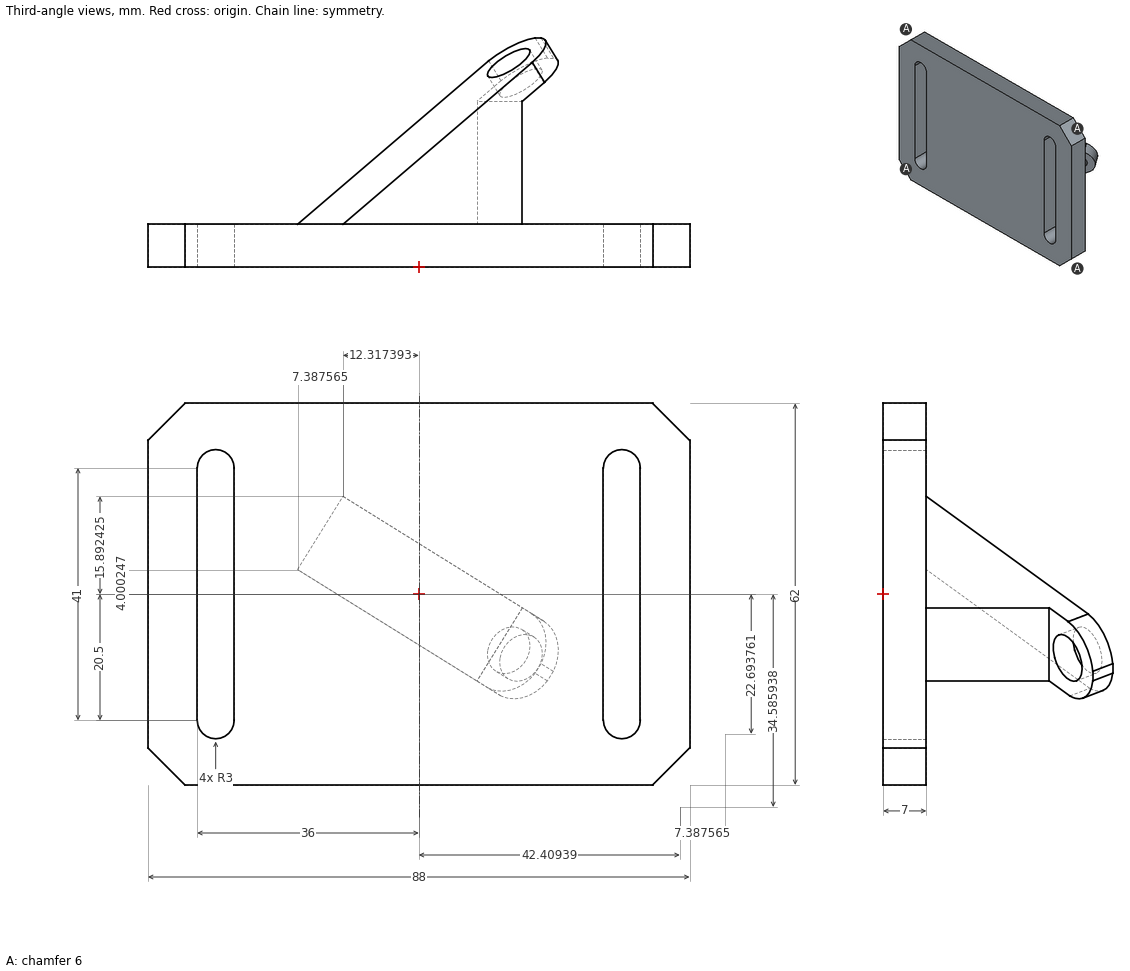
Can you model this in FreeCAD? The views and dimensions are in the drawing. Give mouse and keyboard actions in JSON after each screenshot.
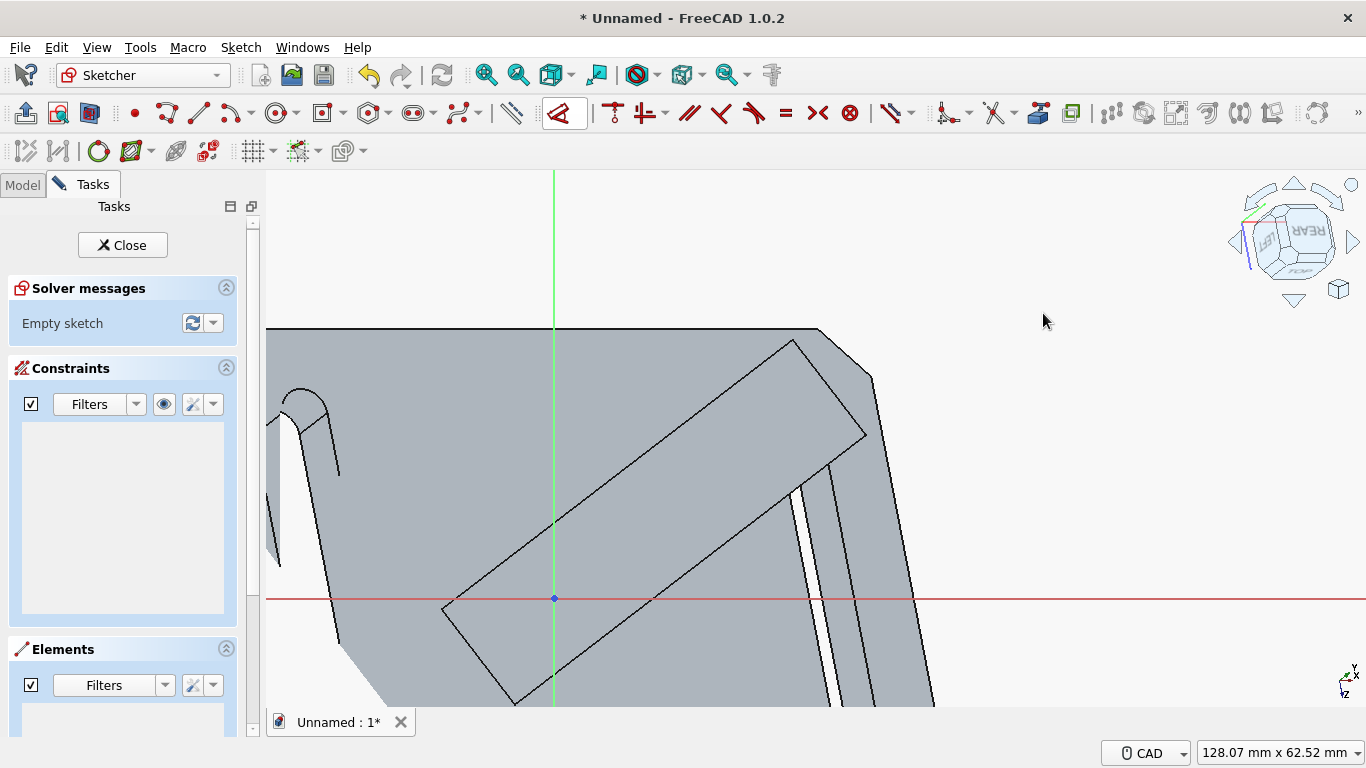
{"action": "left_click", "coordinate": [168, 114]}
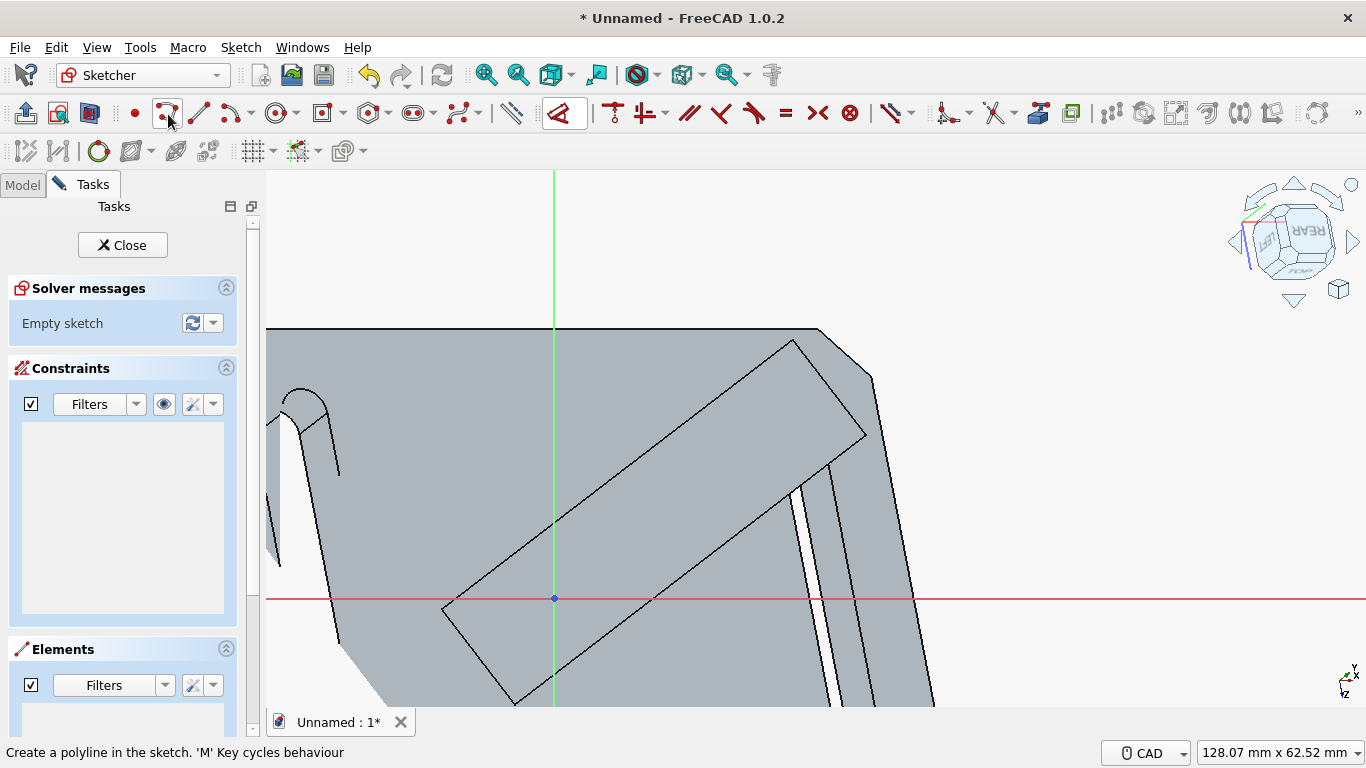
{"action": "left_click", "coordinate": [819, 471]}
{"action": "left_click", "coordinate": [856, 453]}
{"action": "left_click", "coordinate": [939, 464]}
{"action": "left_click", "coordinate": [772, 277]}
{"action": "left_click", "coordinate": [741, 379]}
{"action": "right_click", "coordinate": [741, 379]}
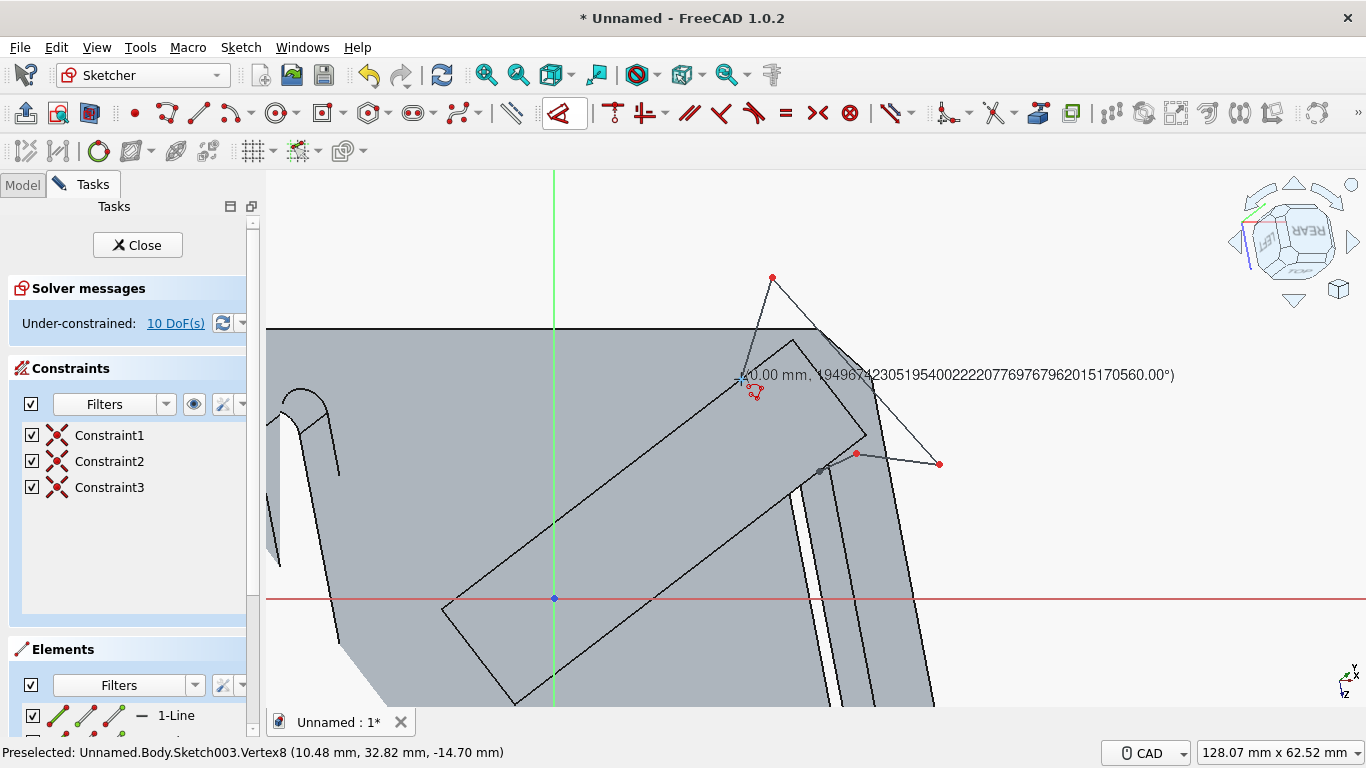
{"action": "left_click", "coordinate": [254, 114]}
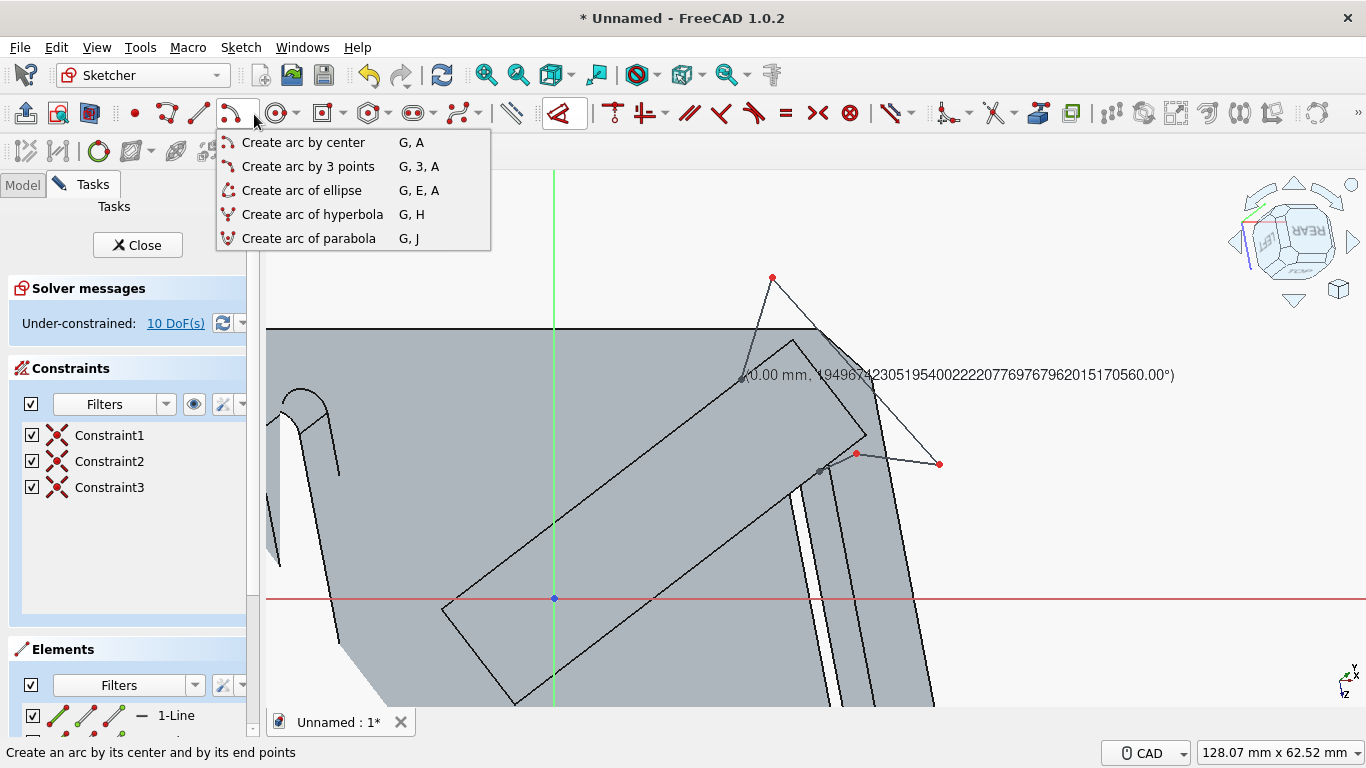
{"action": "left_click", "coordinate": [354, 166]}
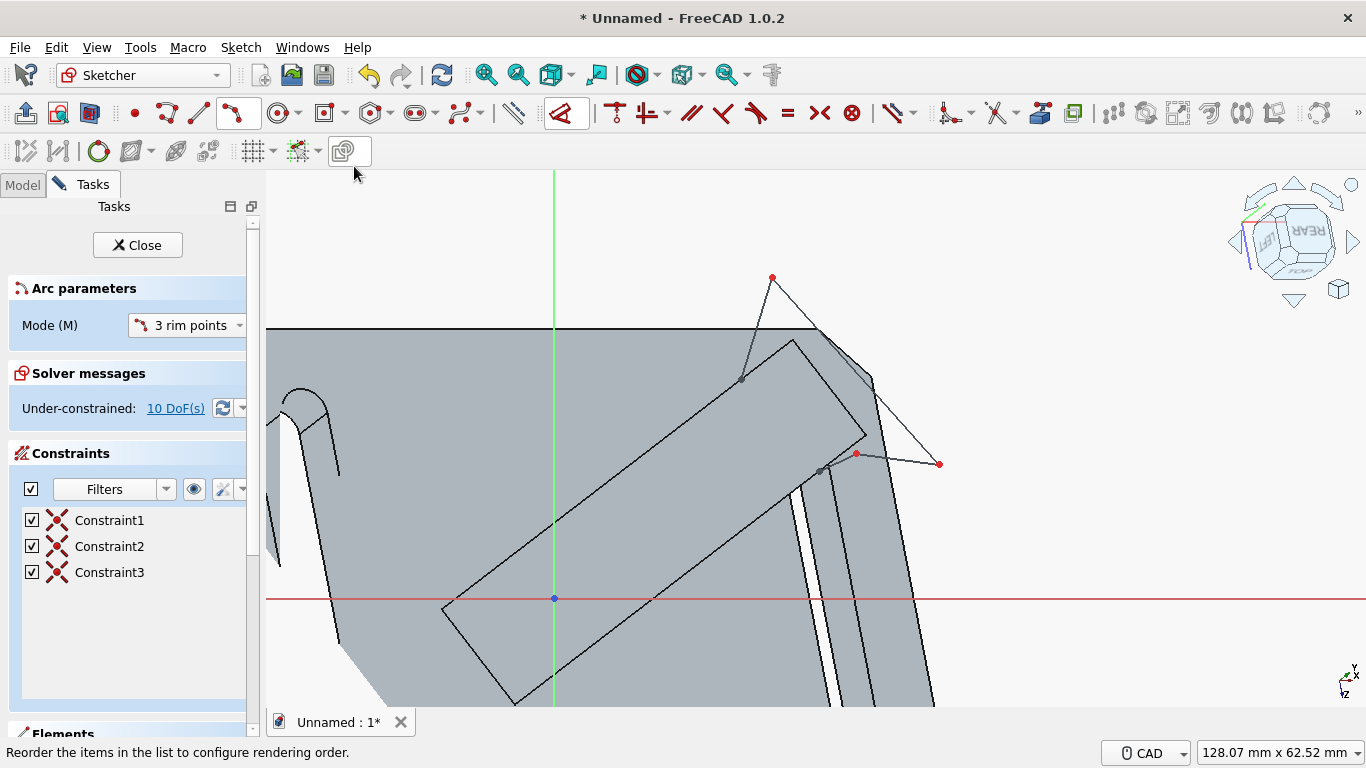
{"action": "left_click", "coordinate": [741, 380]}
{"action": "left_click", "coordinate": [819, 472]}
{"action": "left_click", "coordinate": [828, 385]}
{"action": "key", "text": "Escape"}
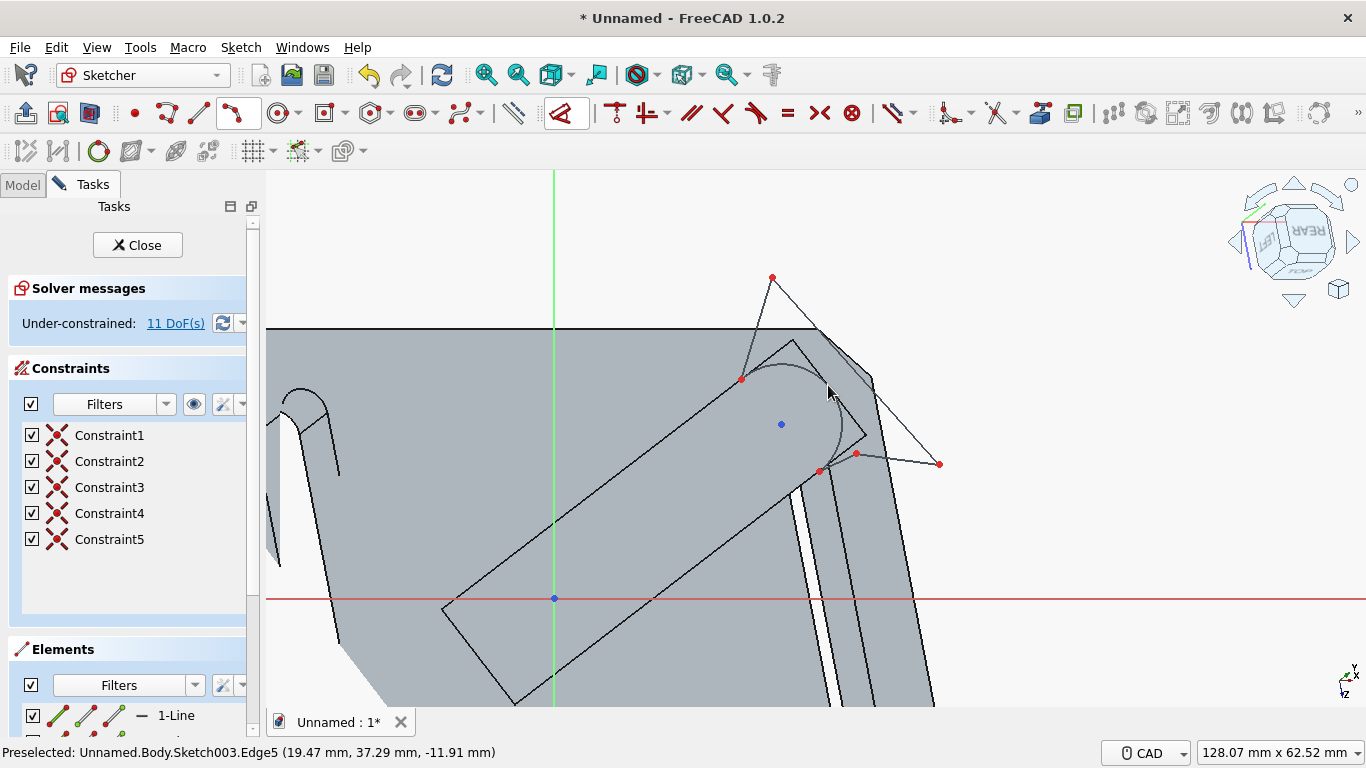
{"action": "left_click", "coordinate": [842, 421]}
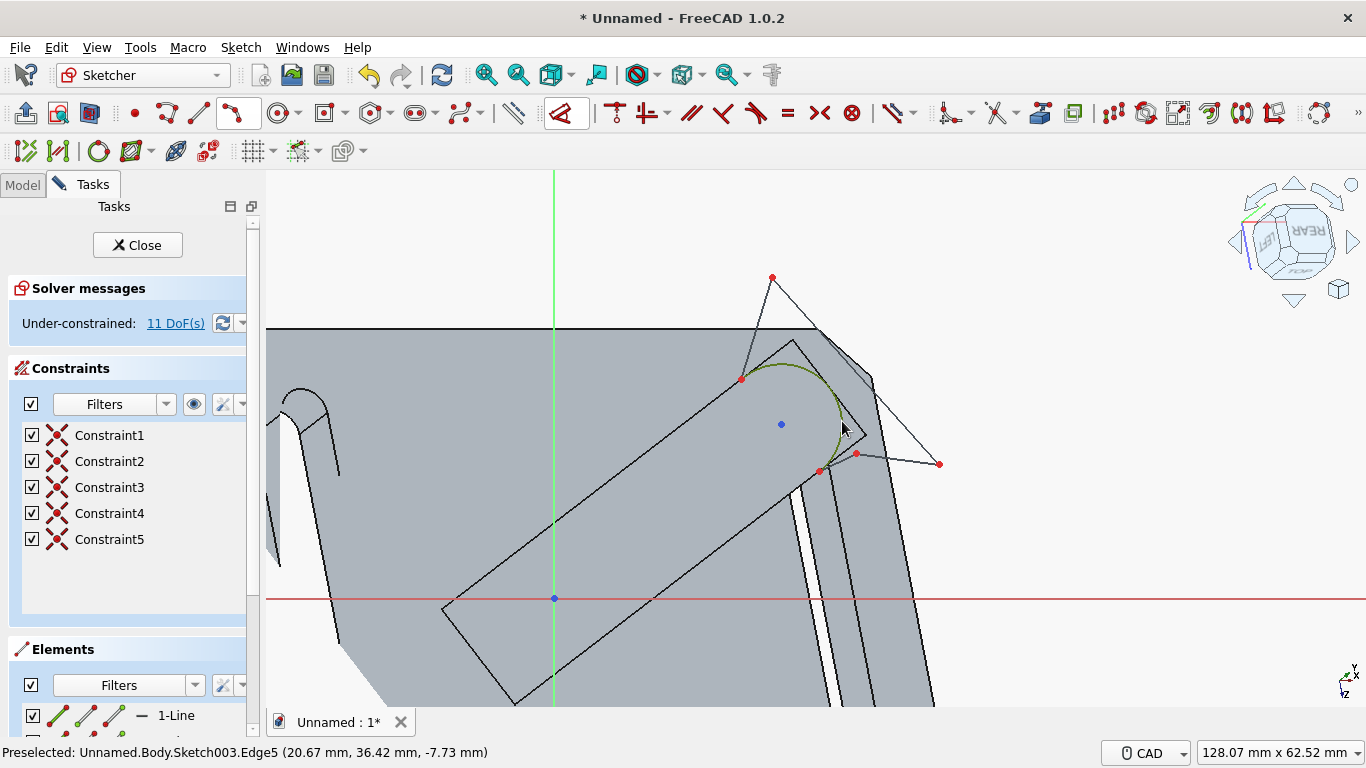
{"action": "left_click", "coordinate": [584, 114]}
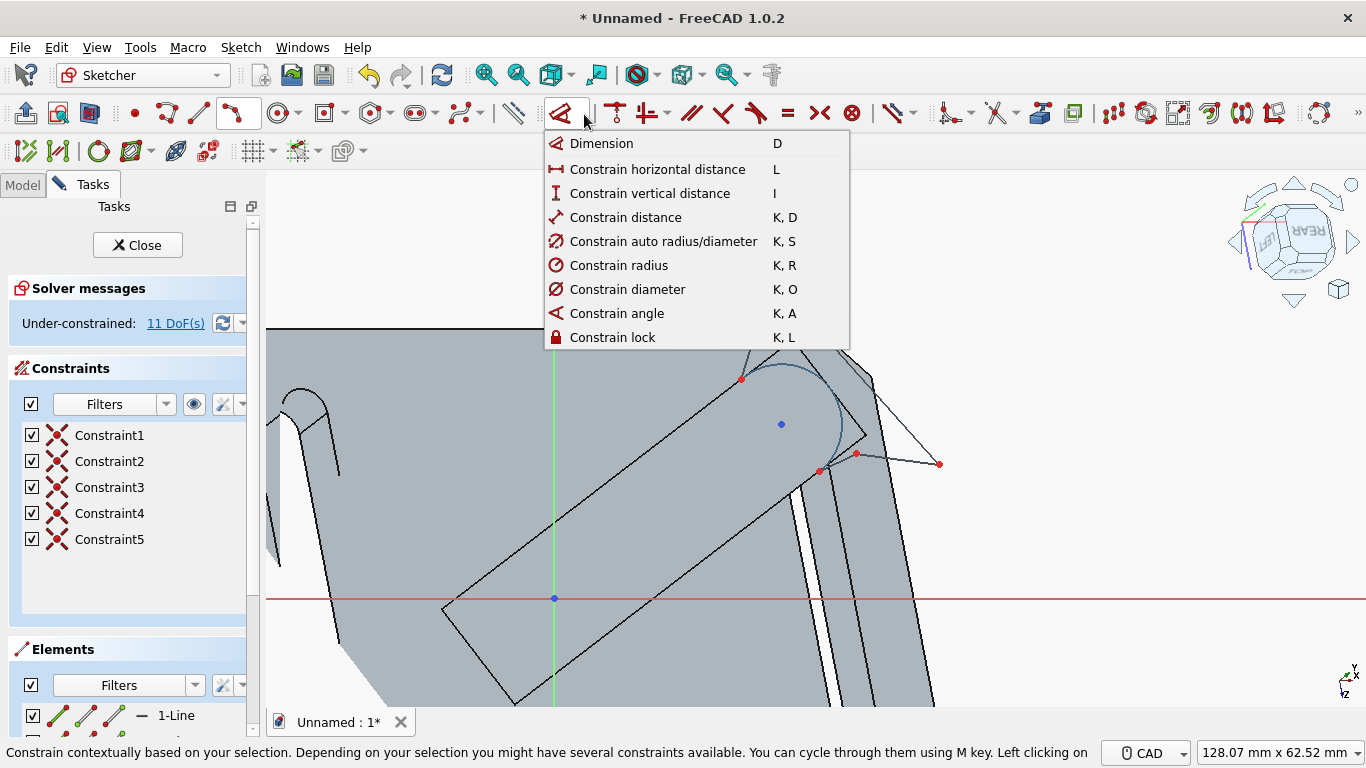
{"action": "left_click", "coordinate": [697, 265]}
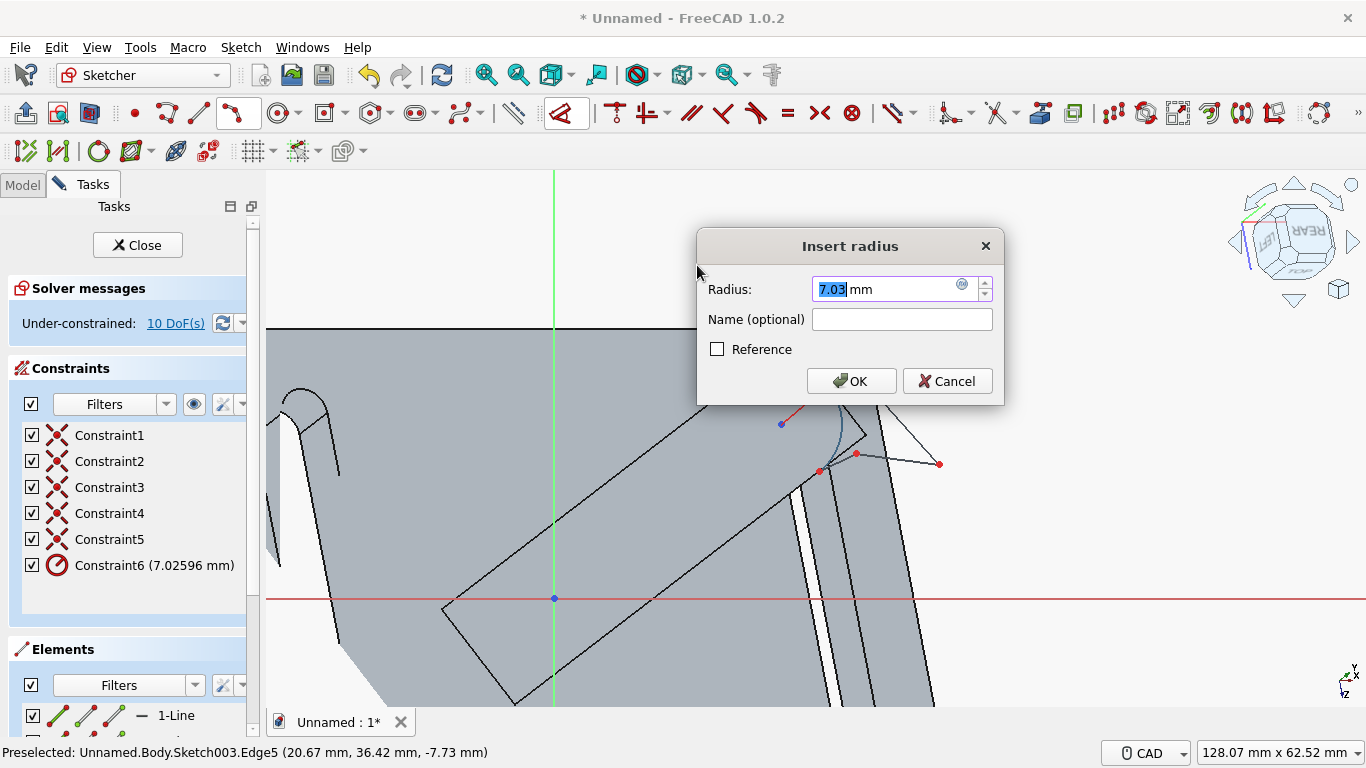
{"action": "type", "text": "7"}
{"action": "key", "text": "Return"}